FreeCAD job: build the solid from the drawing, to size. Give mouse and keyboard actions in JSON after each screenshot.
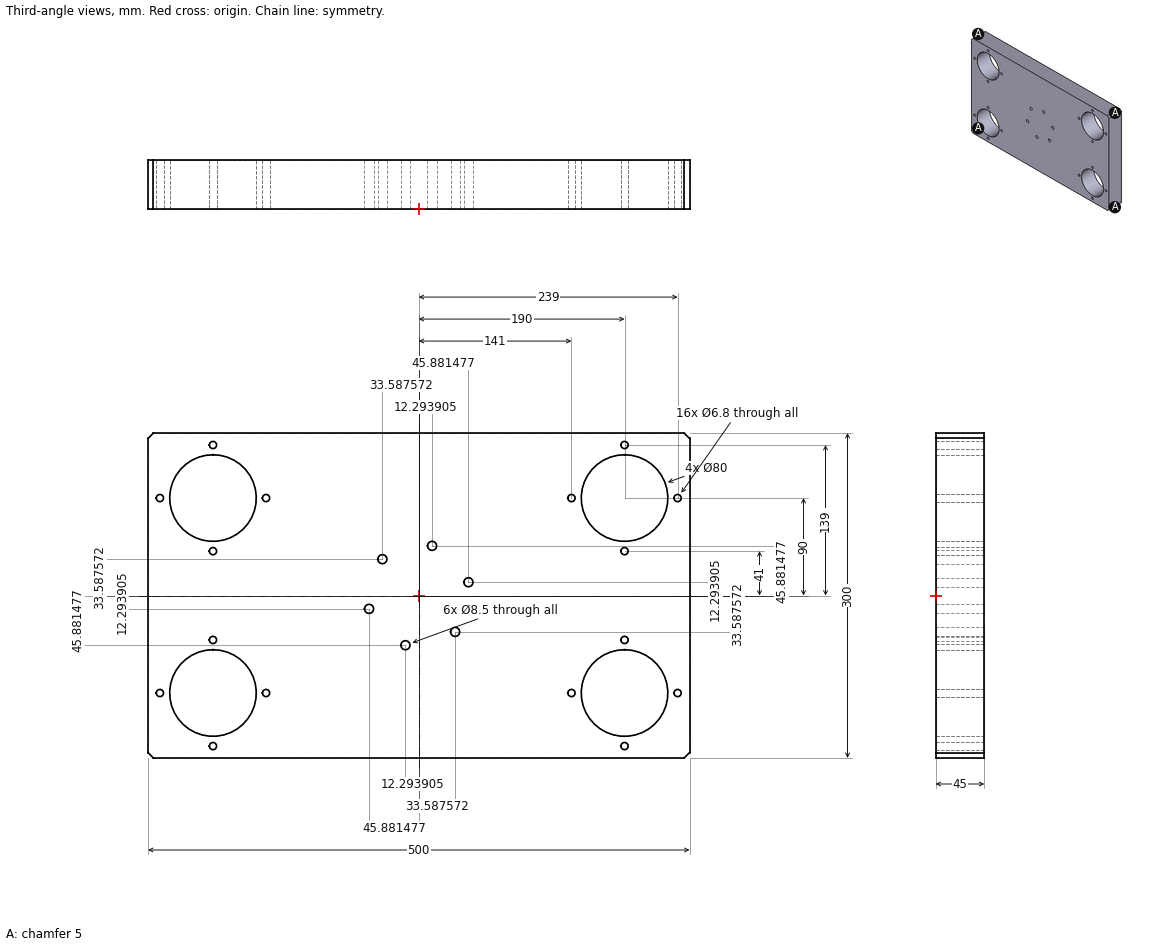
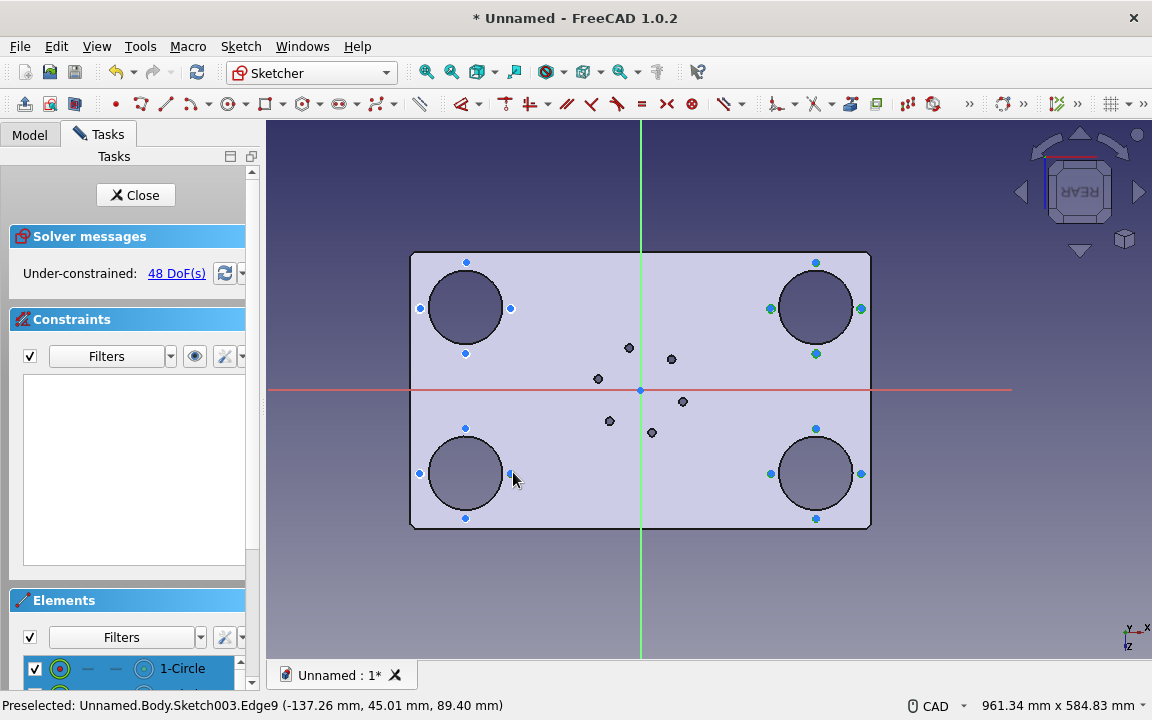
{"action": "scroll", "coordinate": [468, 517], "scroll_direction": "up", "scroll_amount": 8}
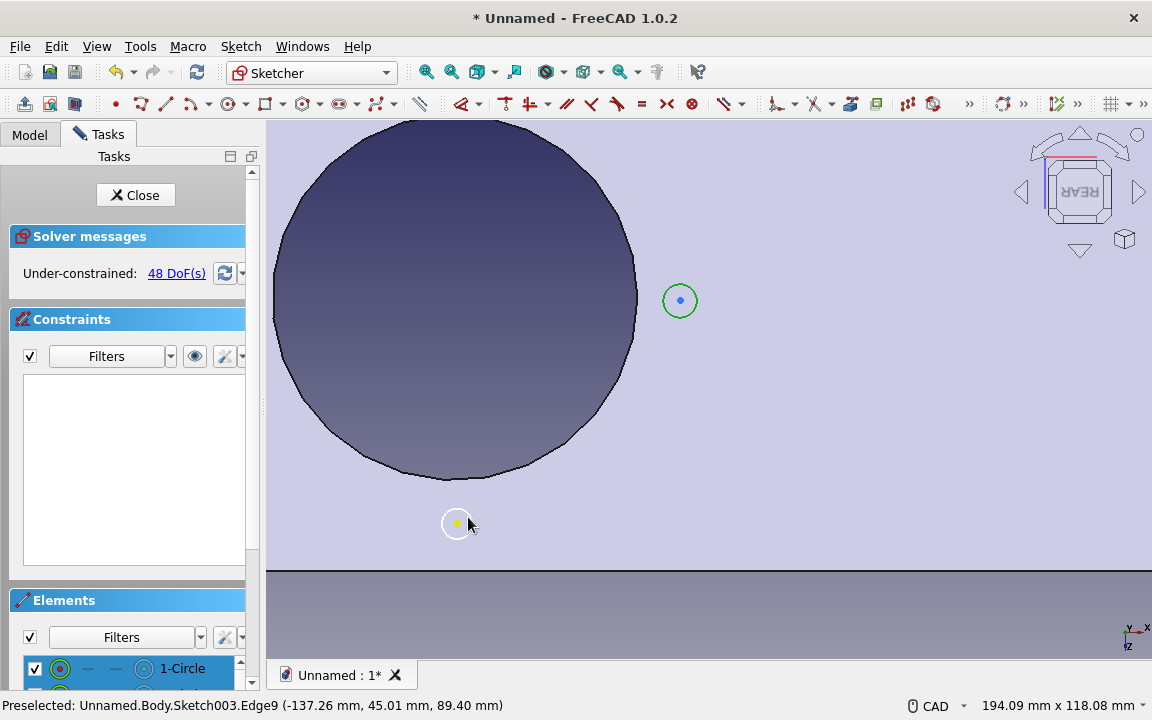
{"action": "left_click", "coordinate": [468, 513]}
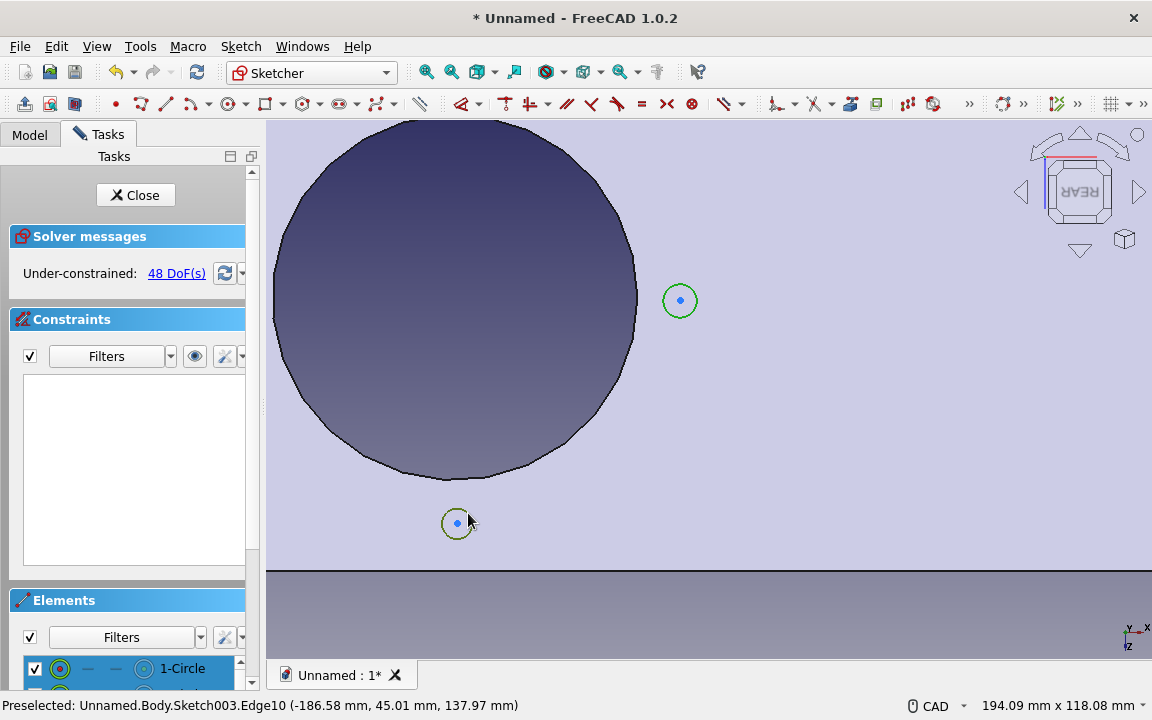
{"action": "scroll", "coordinate": [468, 517], "scroll_direction": "down", "scroll_amount": 8}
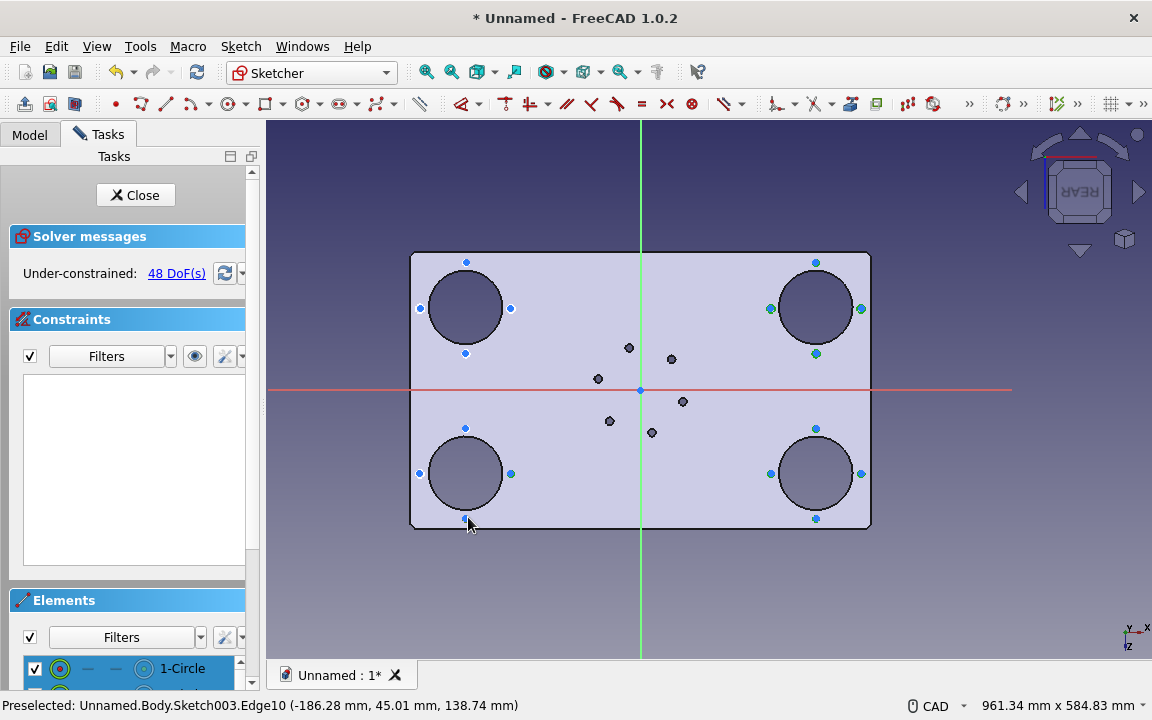
{"action": "scroll", "coordinate": [423, 471], "scroll_direction": "up", "scroll_amount": 7}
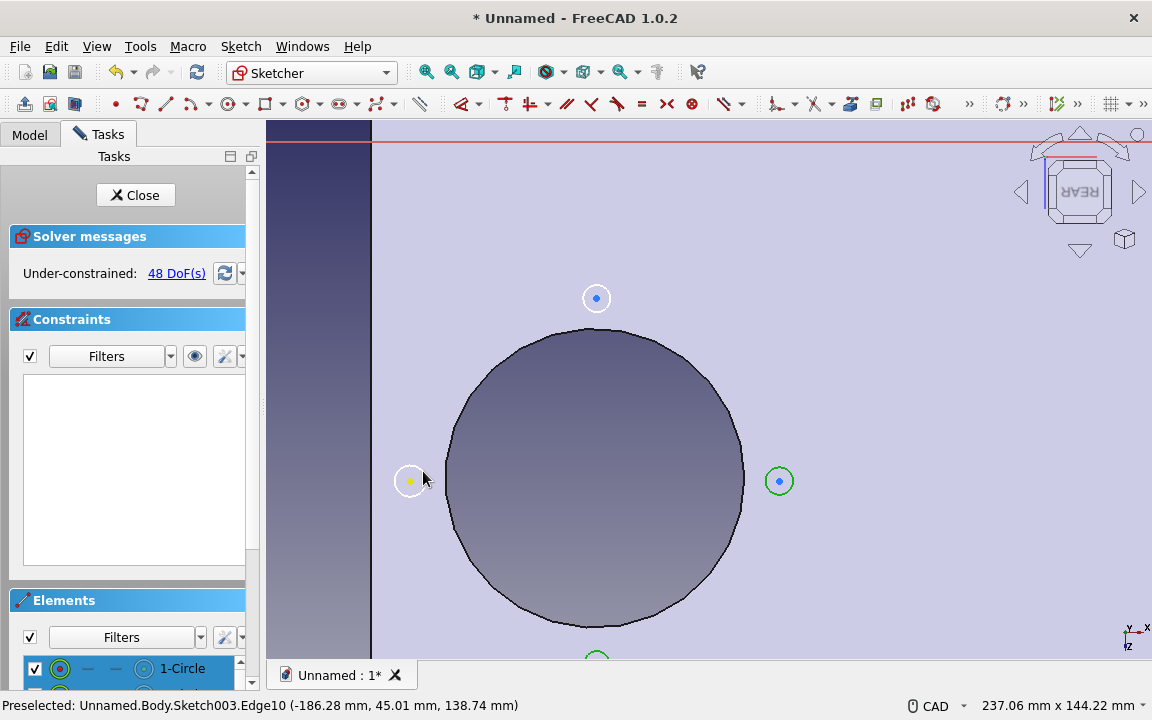
{"action": "left_click", "coordinate": [421, 470]}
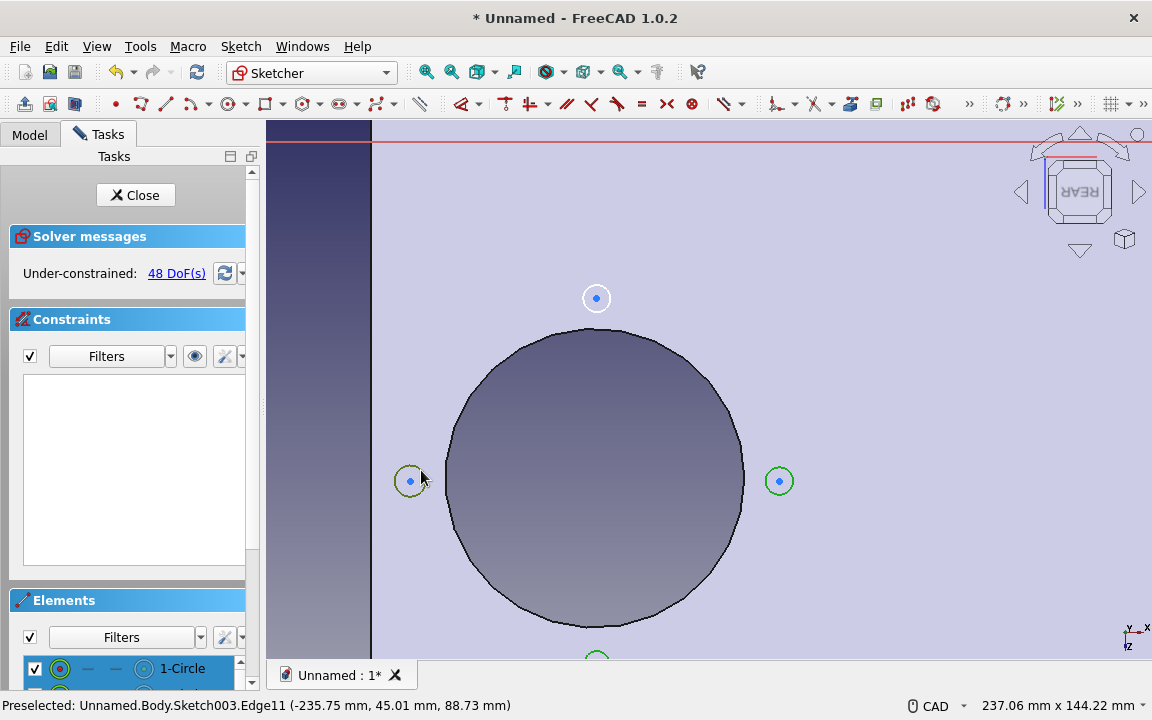
{"action": "left_click", "coordinate": [606, 289]}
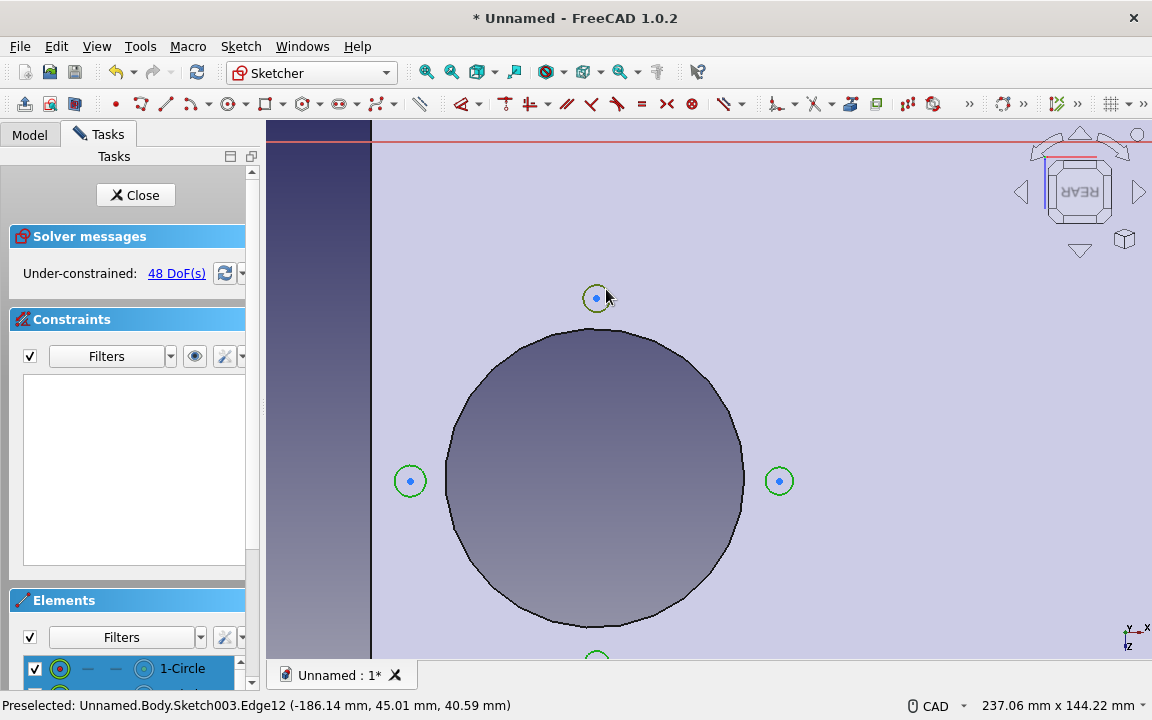
{"action": "scroll", "coordinate": [423, 471], "scroll_direction": "down", "scroll_amount": 7}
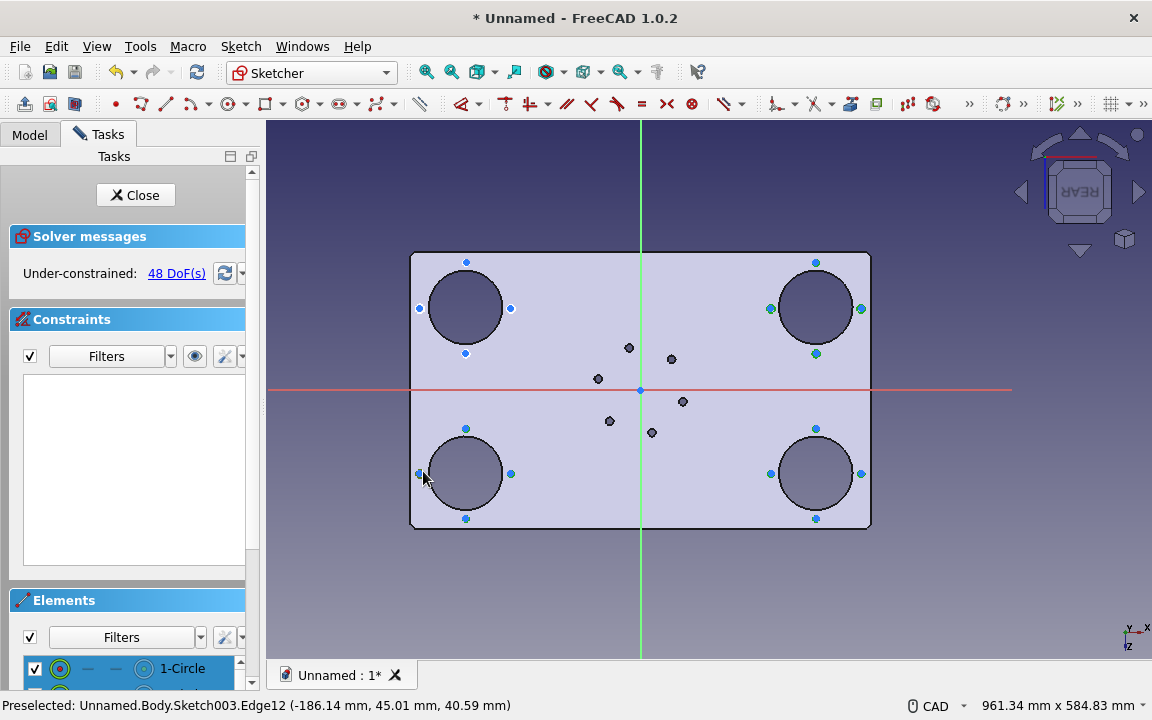
{"action": "scroll", "coordinate": [514, 306], "scroll_direction": "up", "scroll_amount": 7}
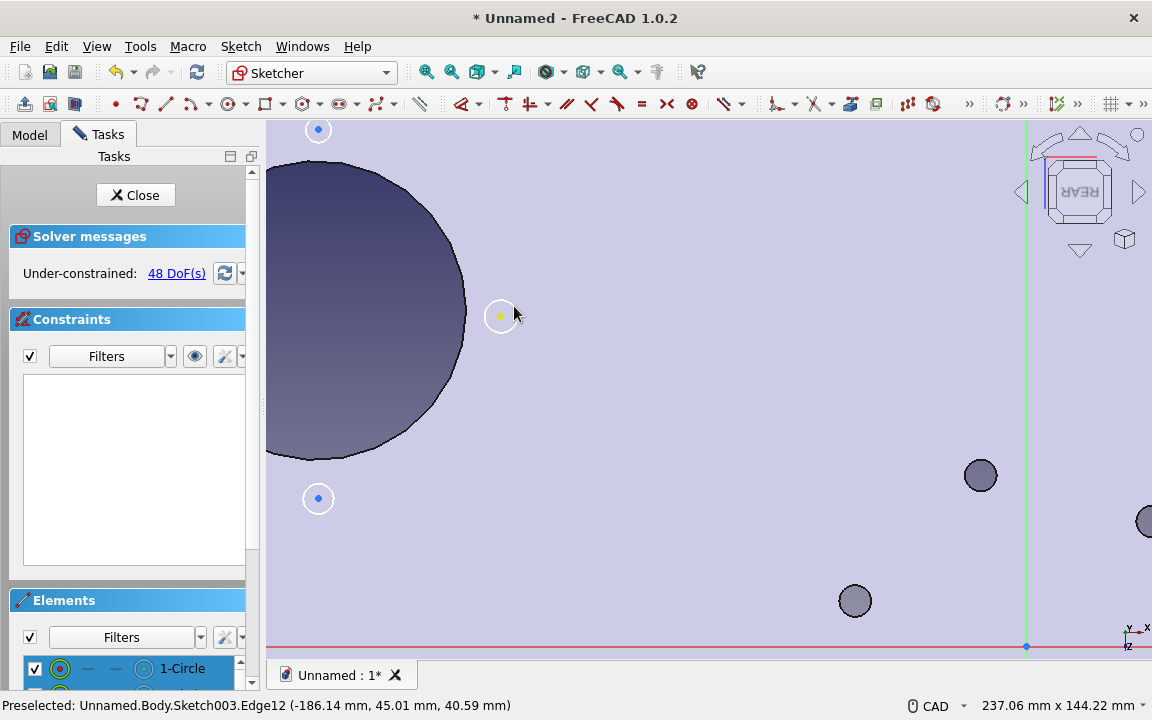
{"action": "left_click", "coordinate": [512, 305]}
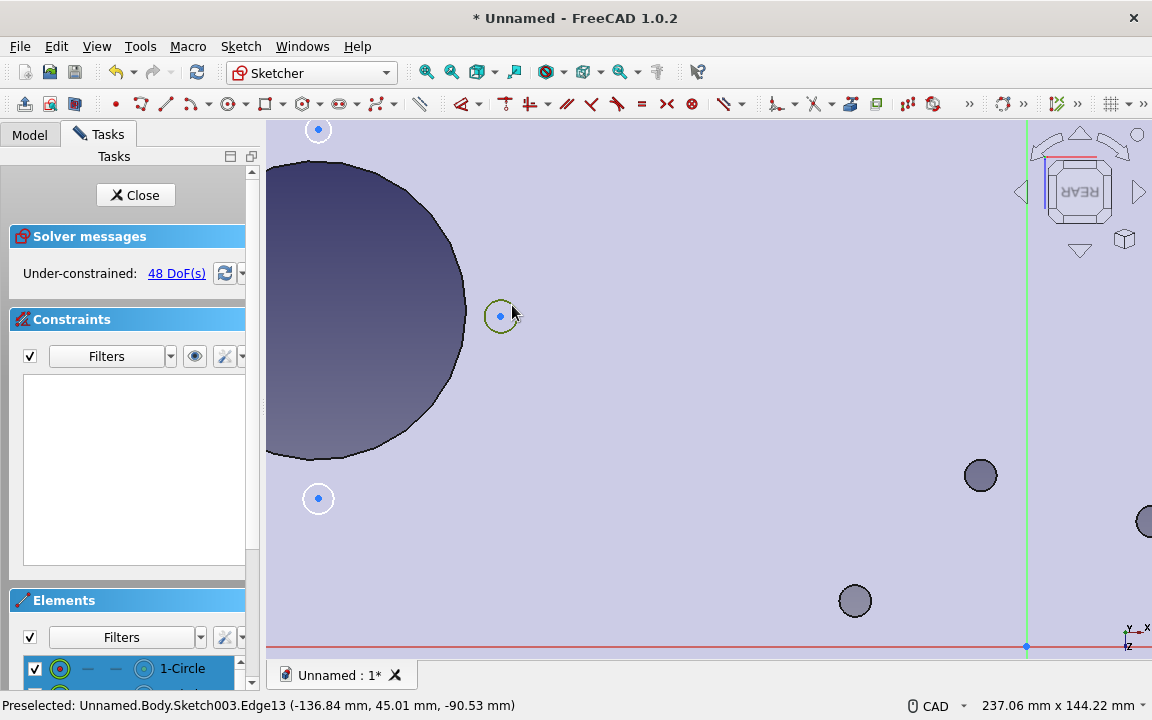
{"action": "left_click", "coordinate": [329, 488]}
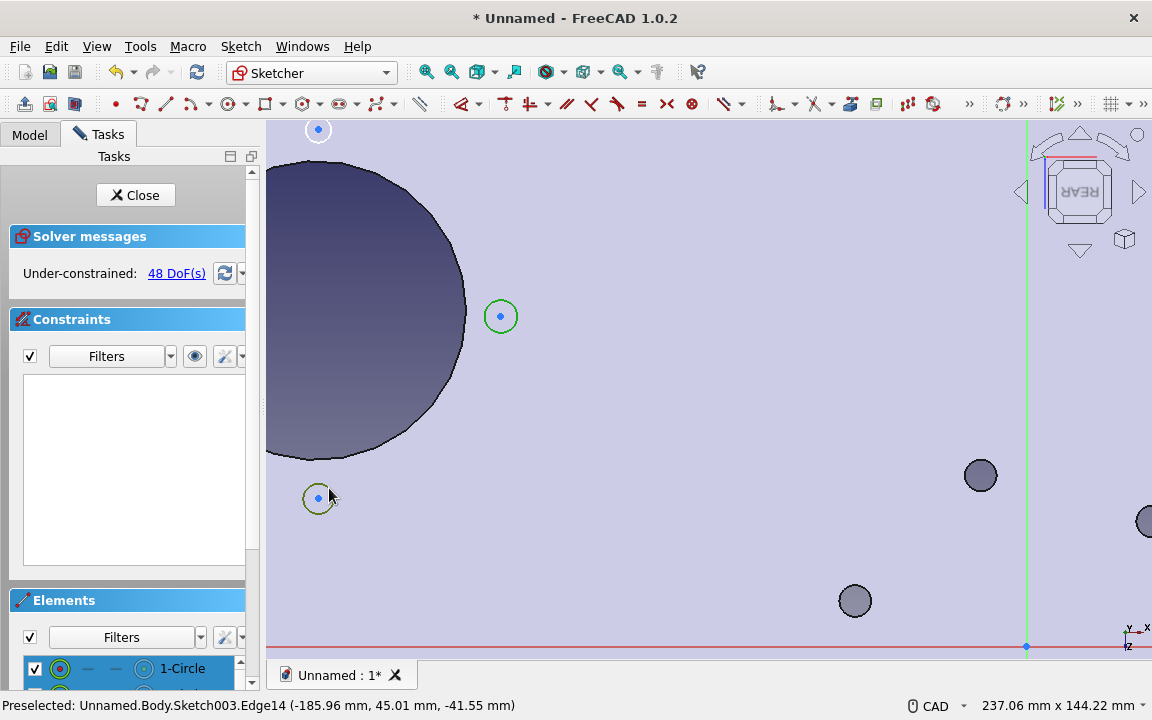
{"action": "scroll", "coordinate": [514, 305], "scroll_direction": "down", "scroll_amount": 7}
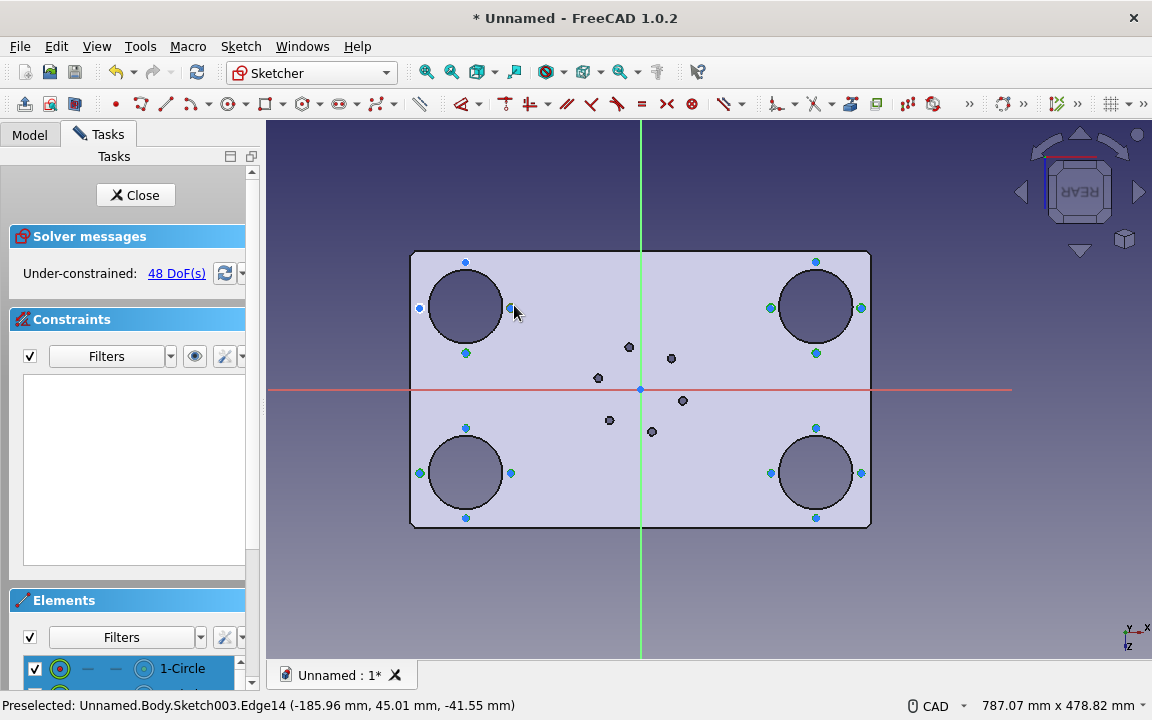
{"action": "scroll", "coordinate": [423, 305], "scroll_direction": "up", "scroll_amount": 6}